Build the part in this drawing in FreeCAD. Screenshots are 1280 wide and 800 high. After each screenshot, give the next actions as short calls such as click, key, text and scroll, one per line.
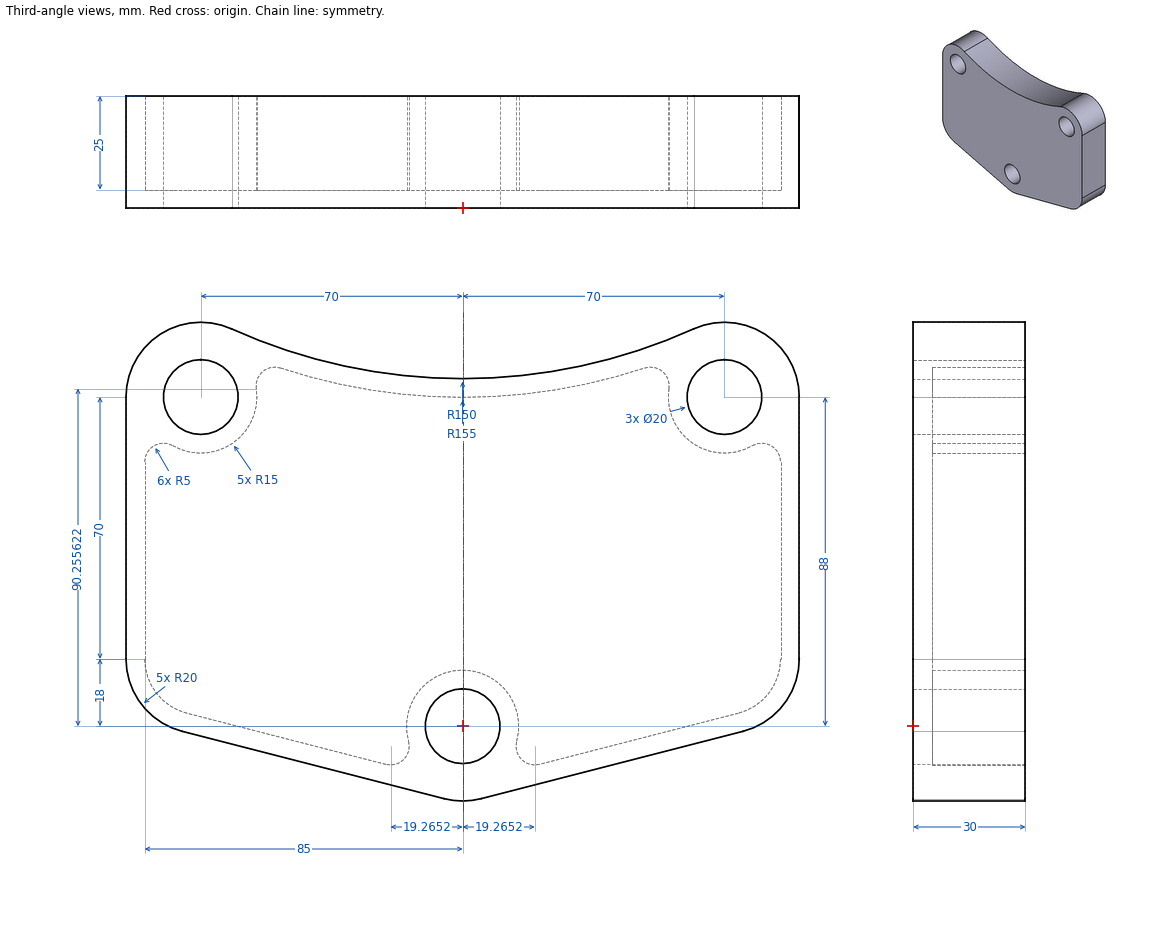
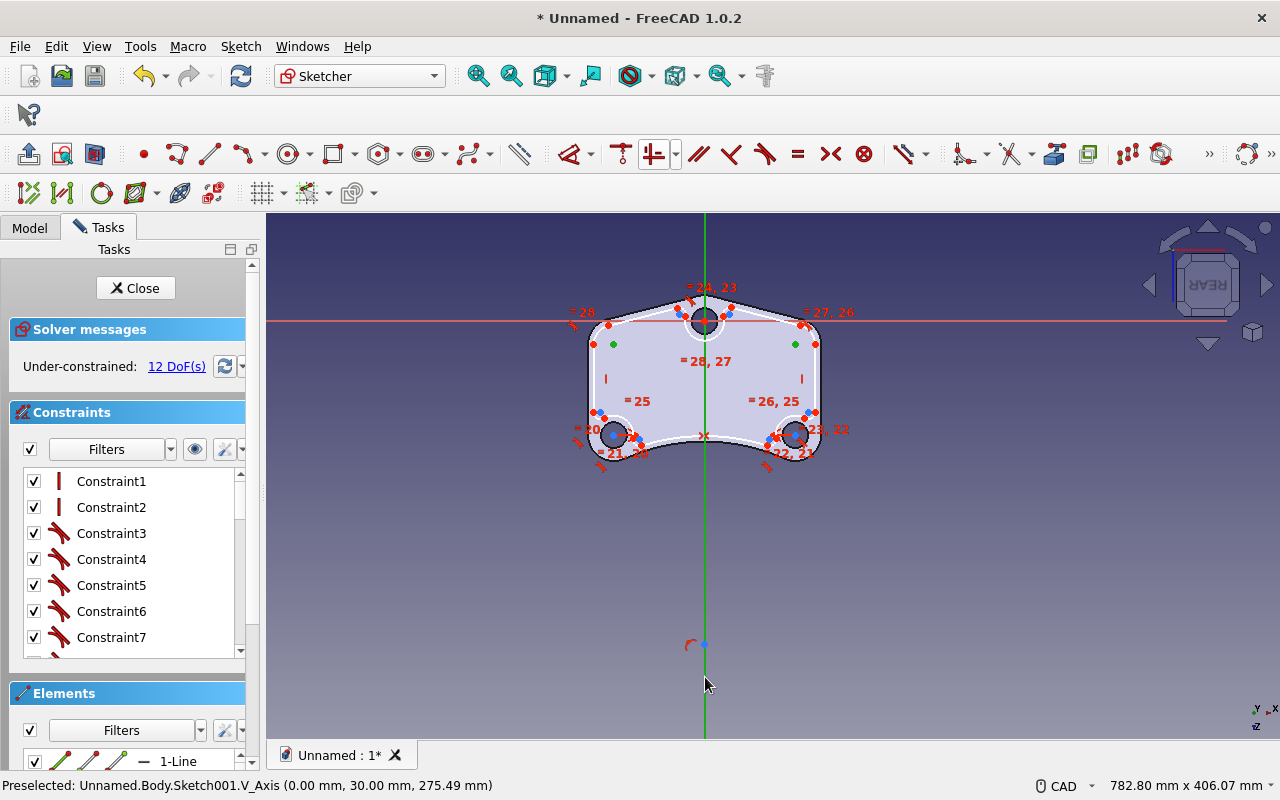
click(831, 154)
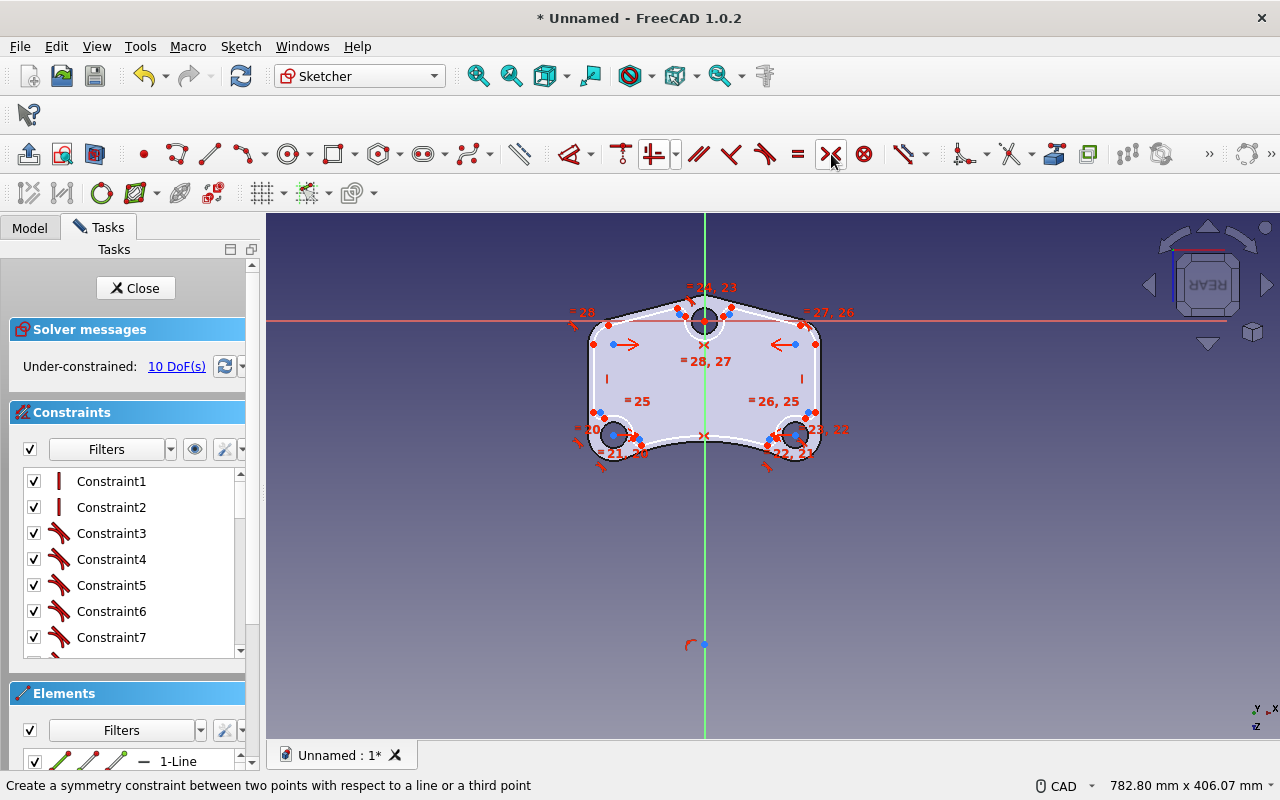
click(568, 154)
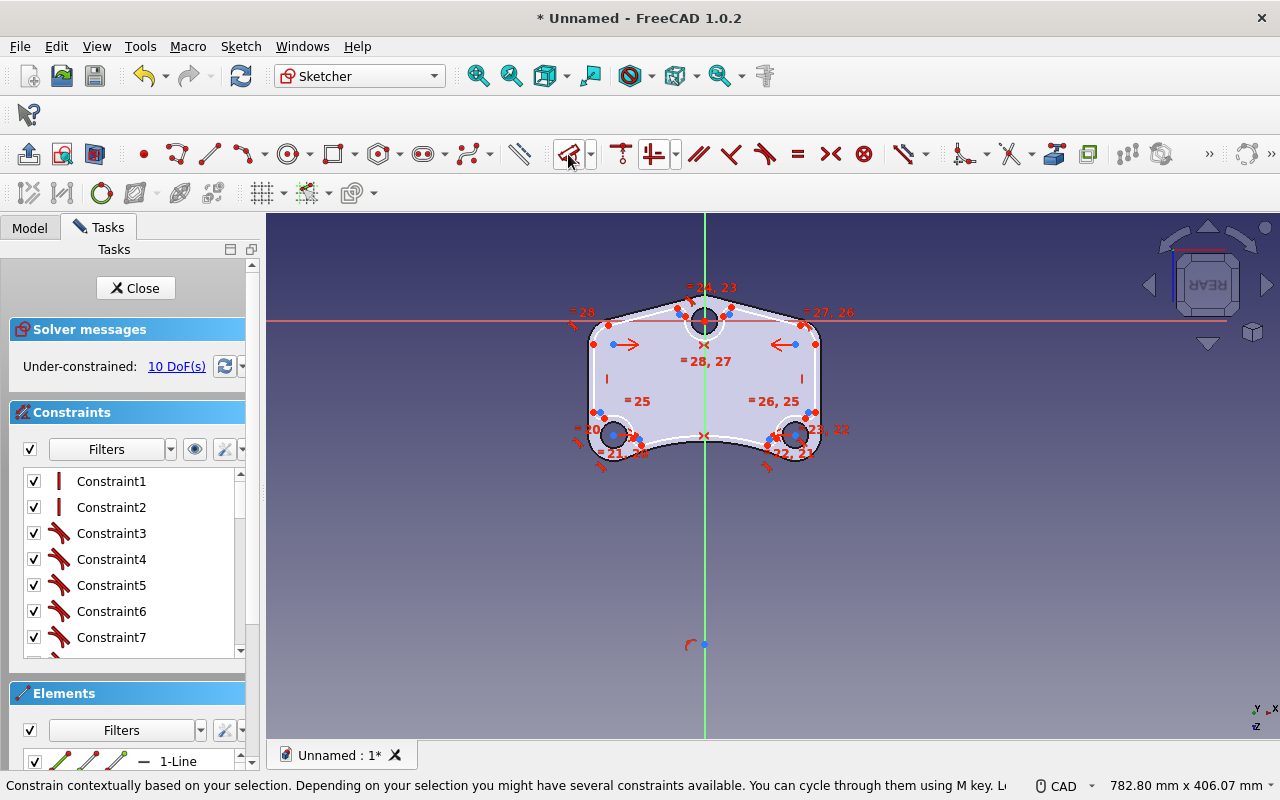
scroll(597, 418, up, 10)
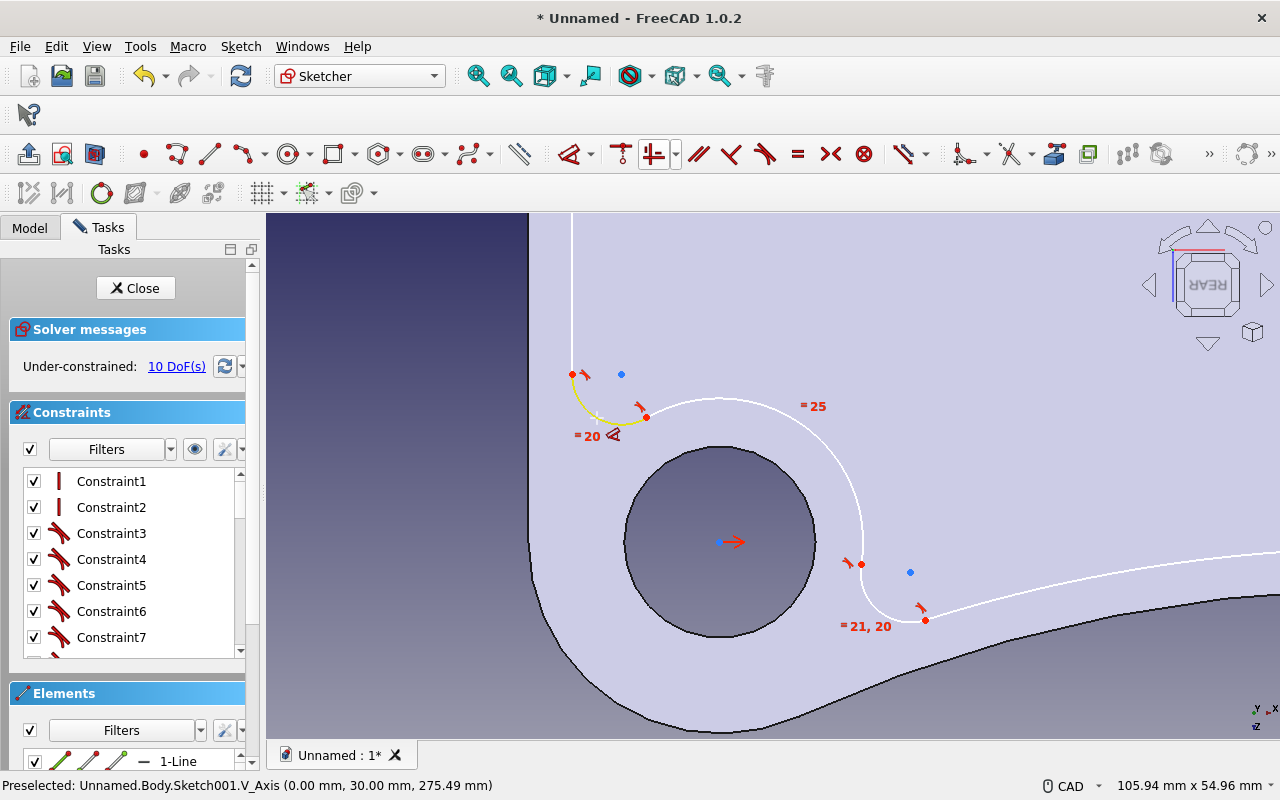
click(597, 418)
click(581, 446)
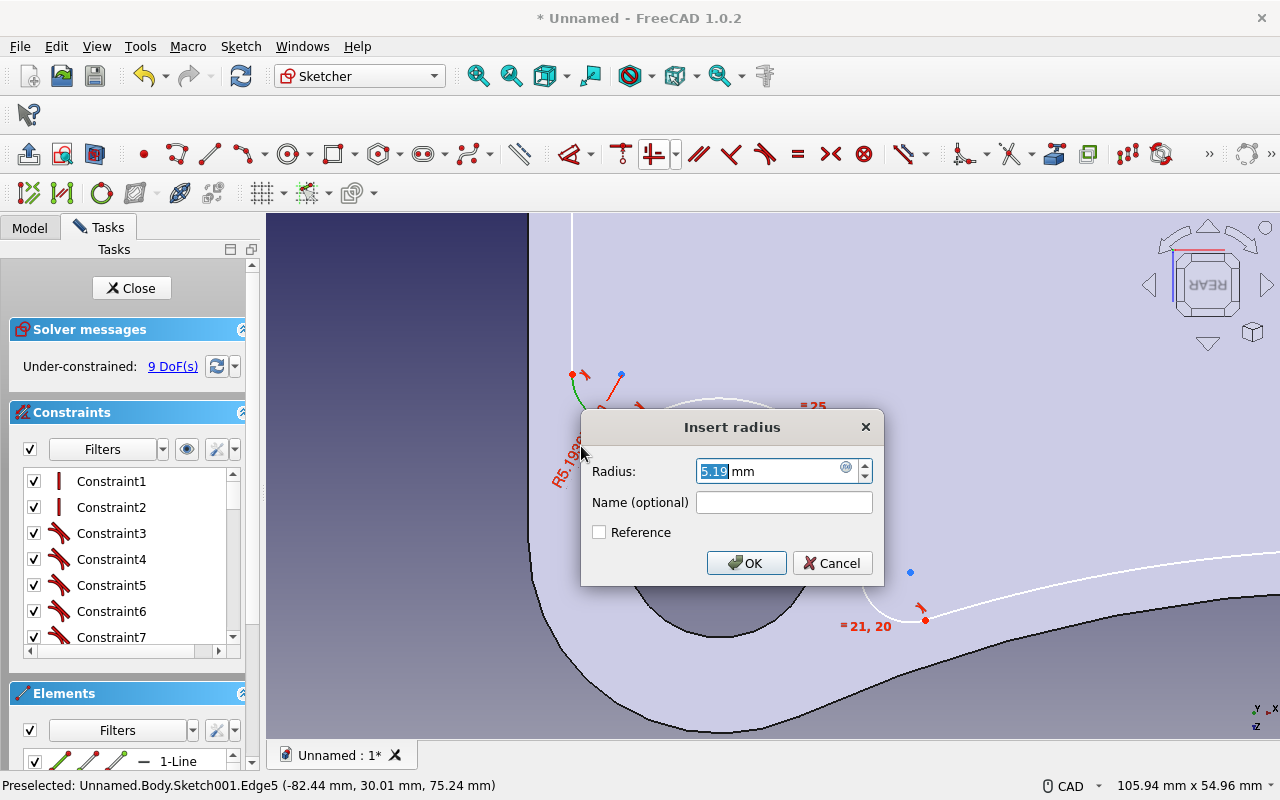
text(5)
key(Return)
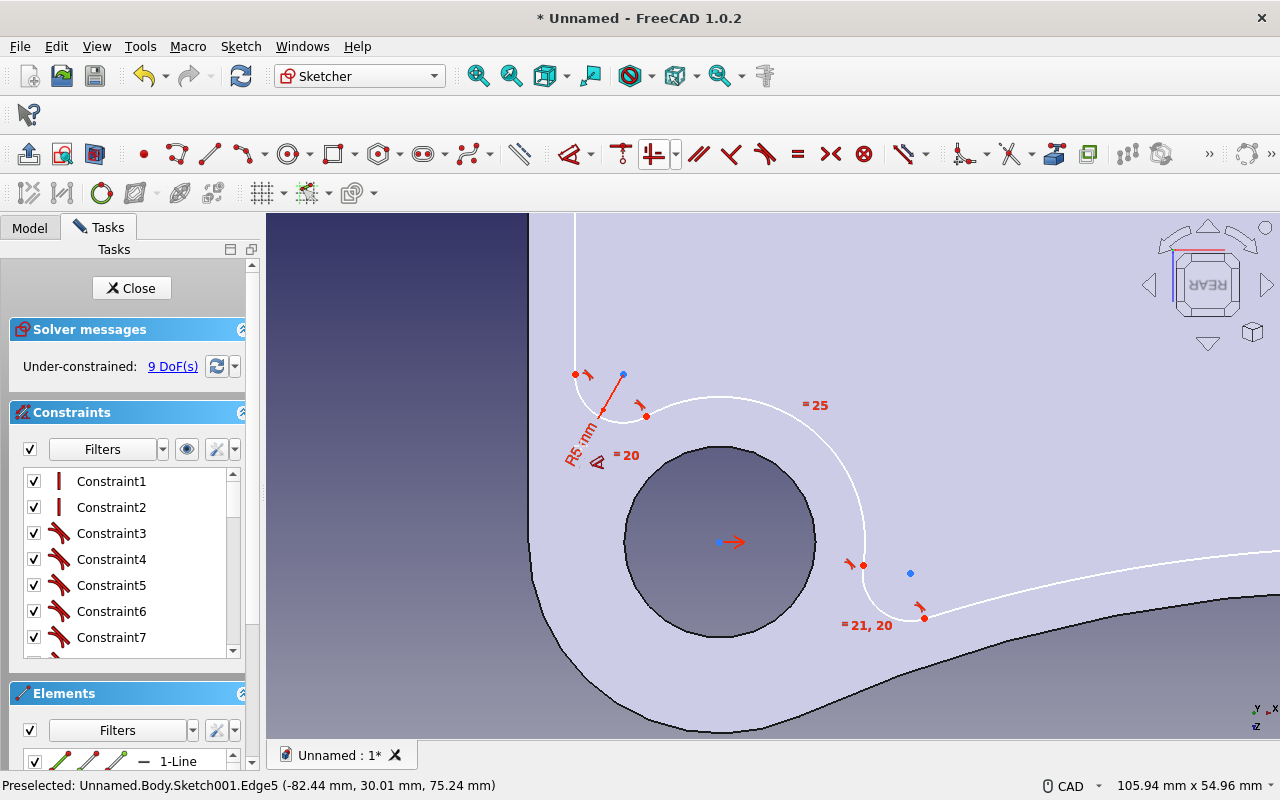
scroll(409, 634, down, 6)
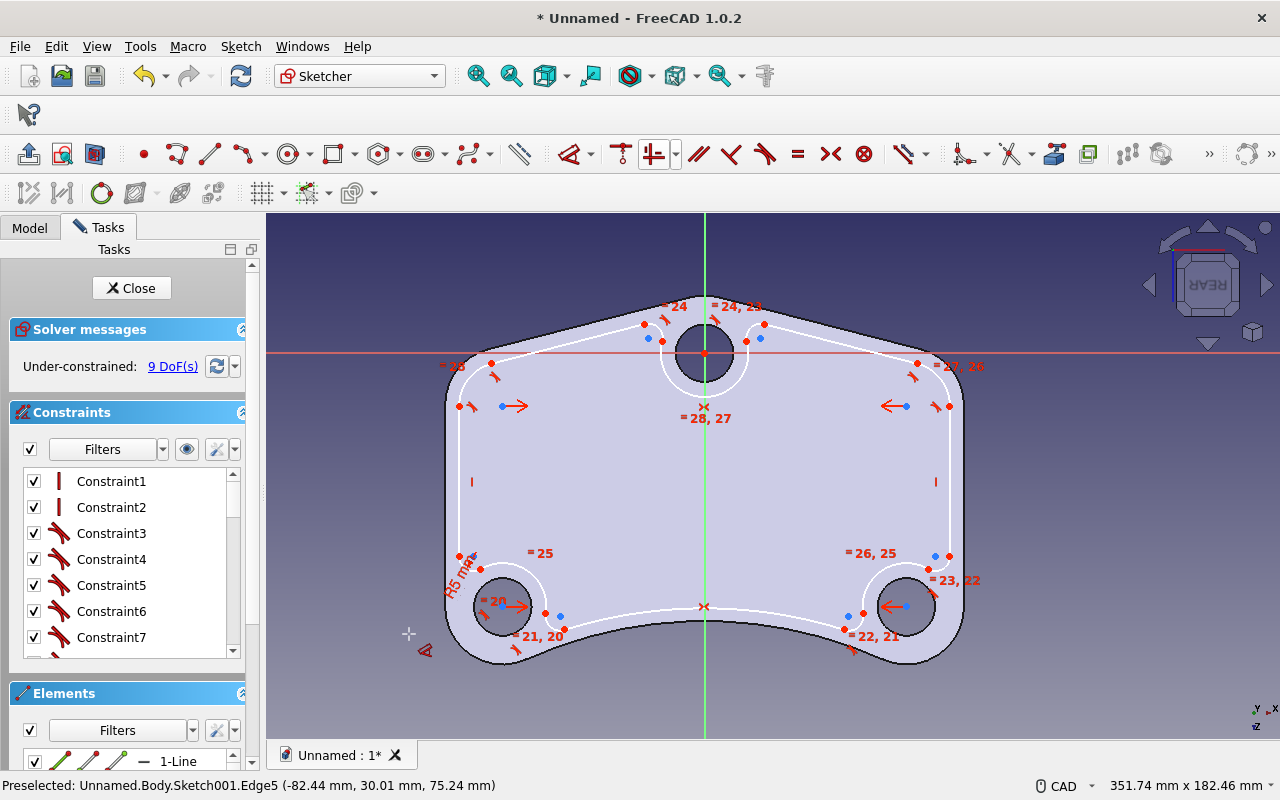
click(541, 585)
click(569, 569)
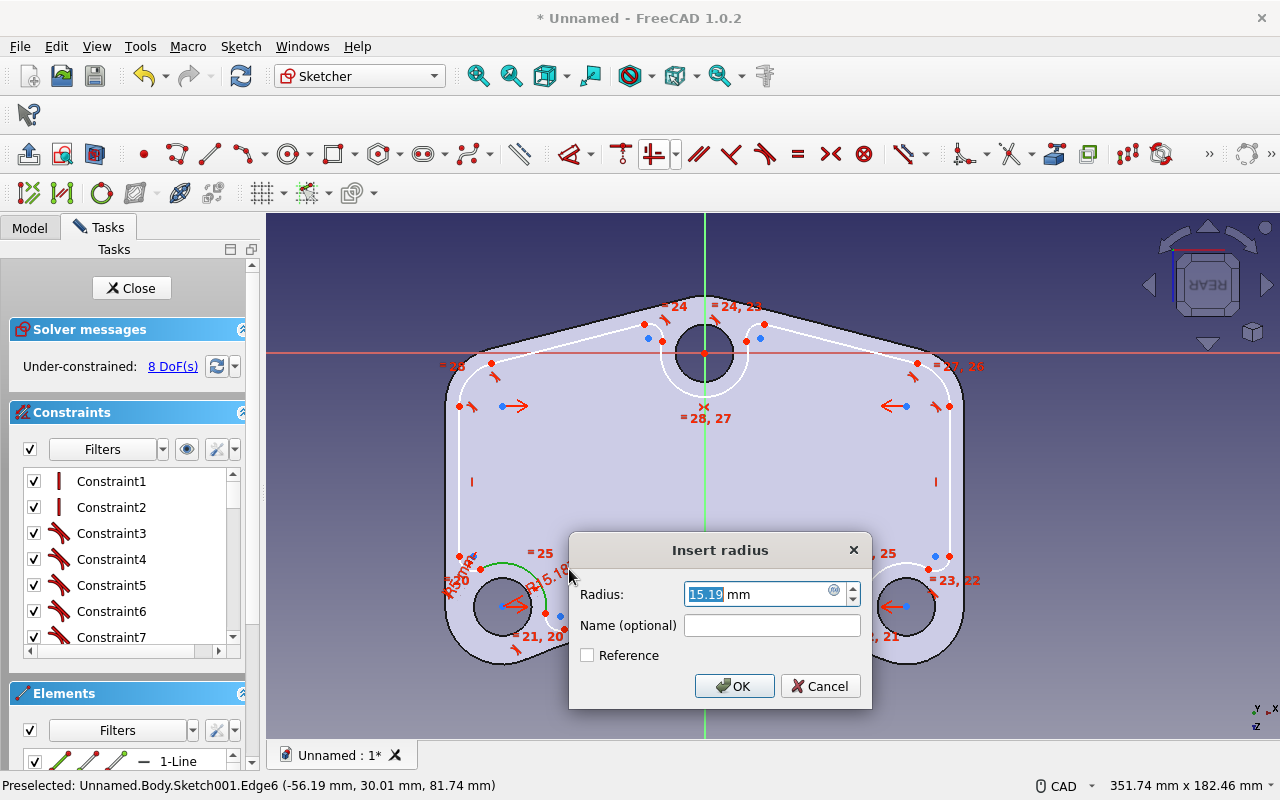
text(15)
key(Return)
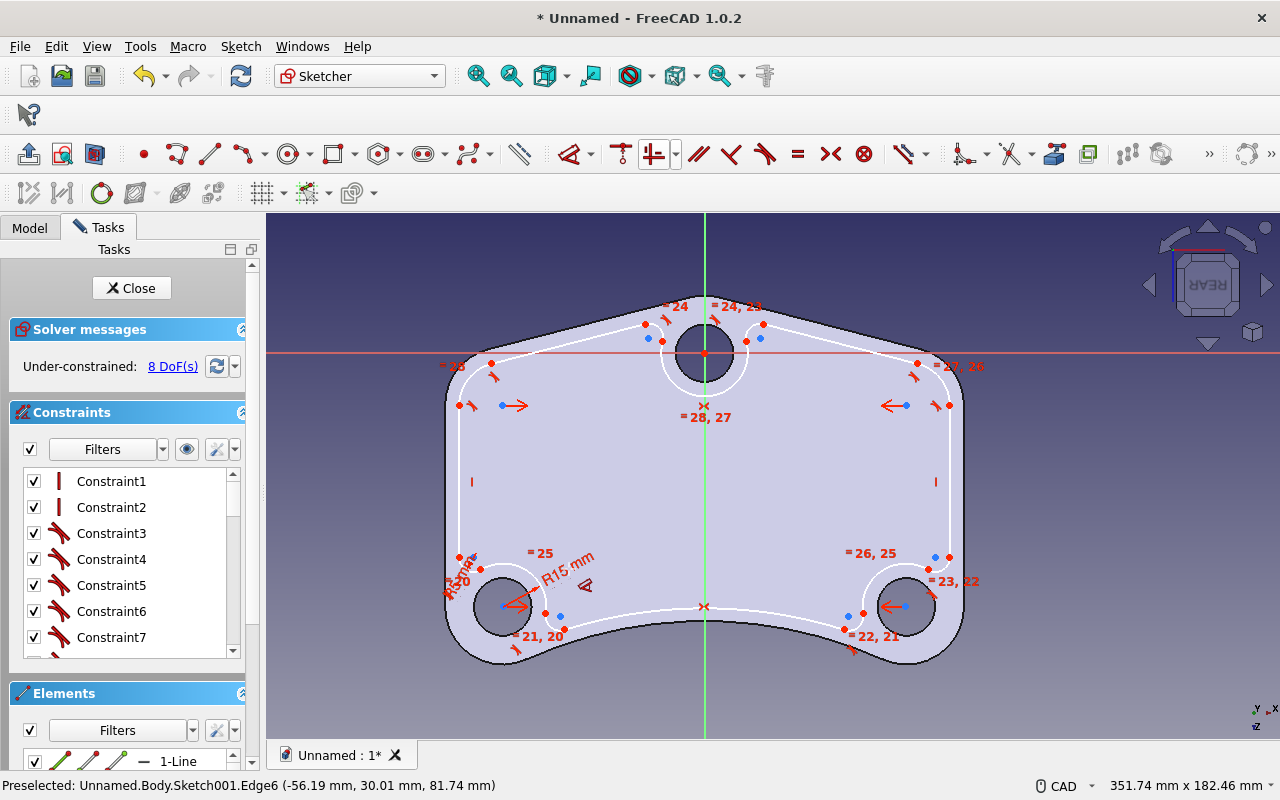
click(761, 612)
click(765, 580)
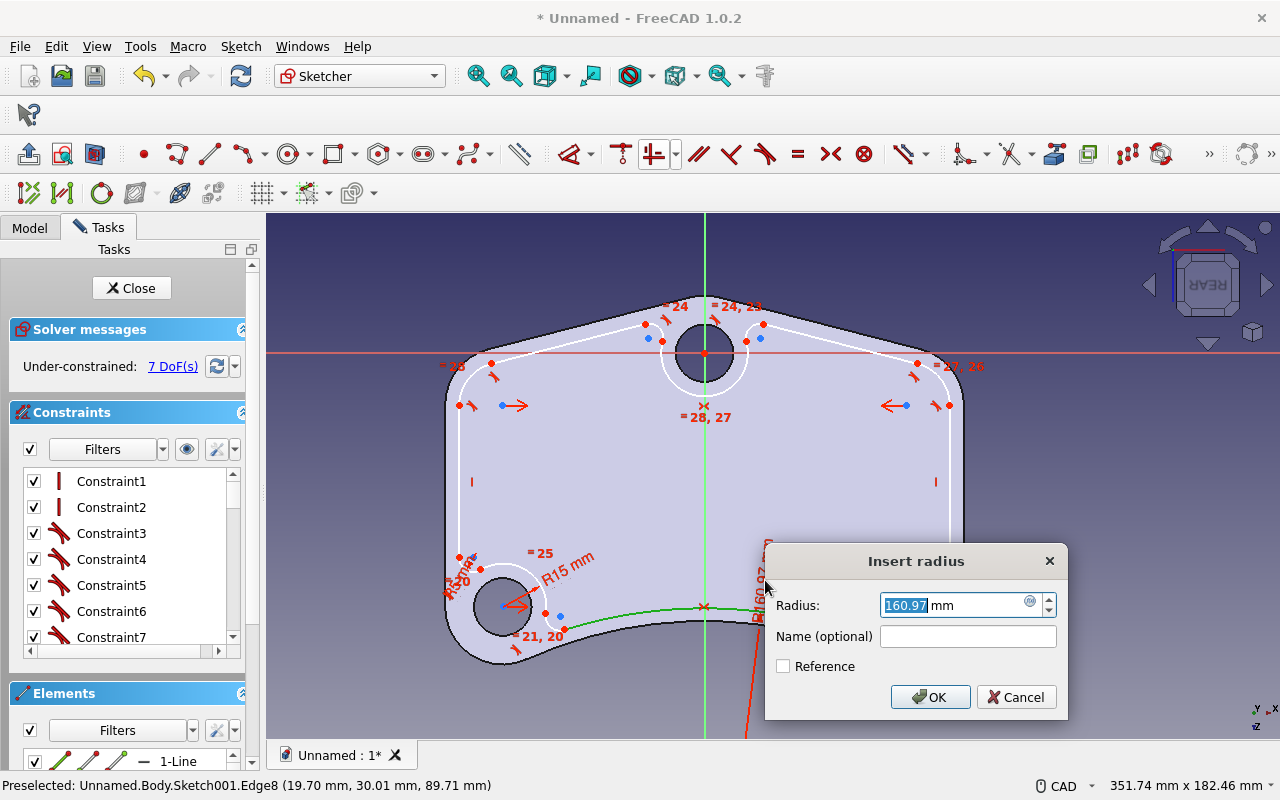
text(155)
key(Return)